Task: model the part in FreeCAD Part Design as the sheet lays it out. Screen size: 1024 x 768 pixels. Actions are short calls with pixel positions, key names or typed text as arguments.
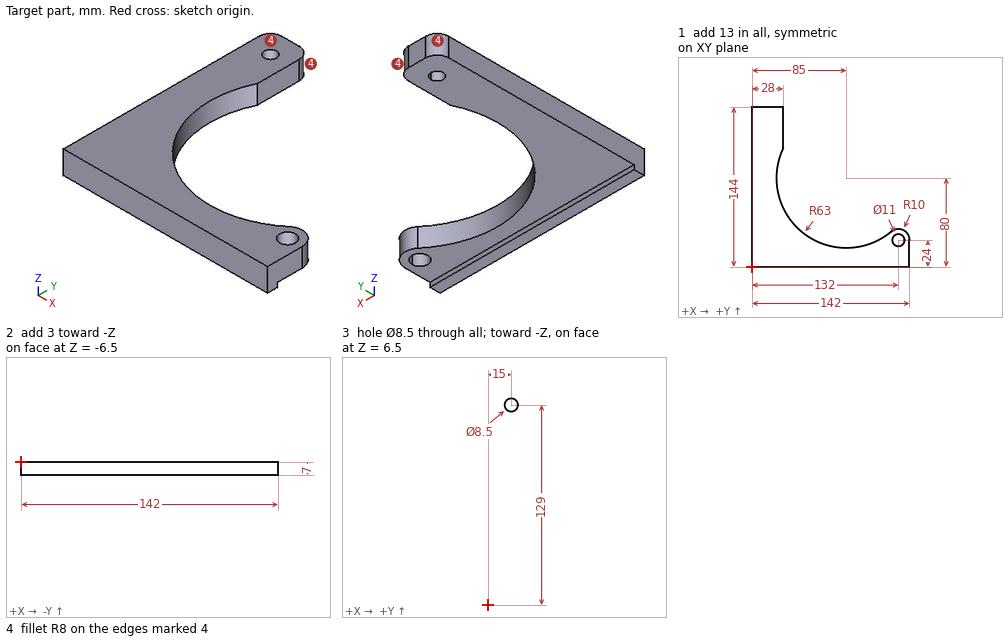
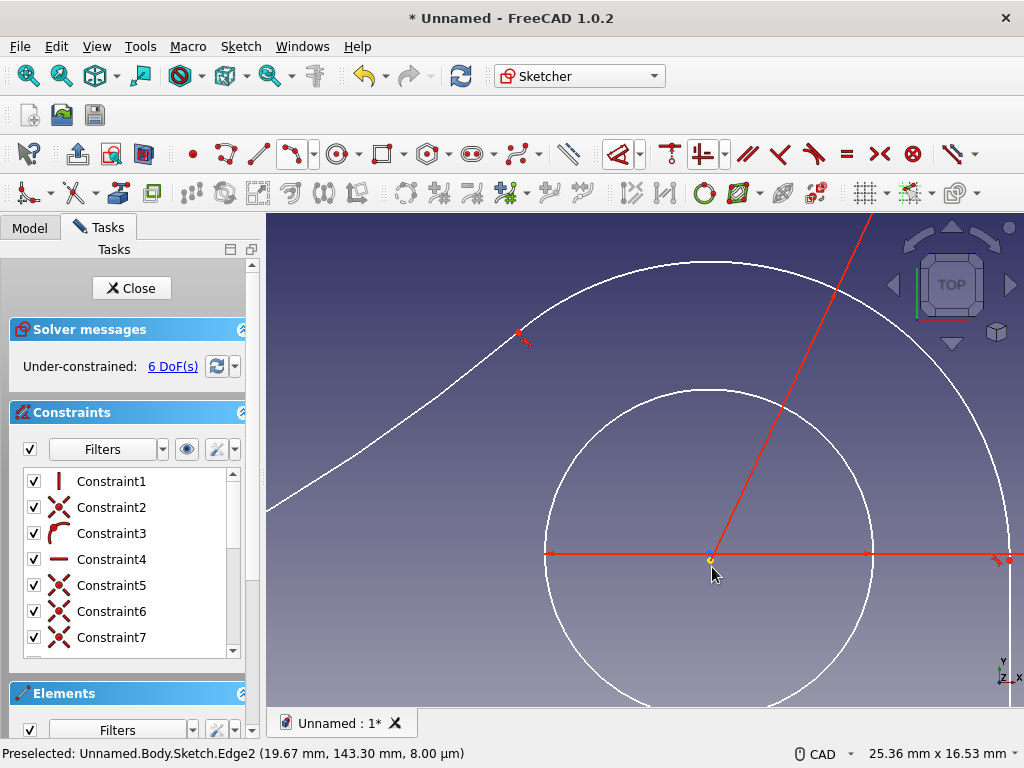
click(709, 554)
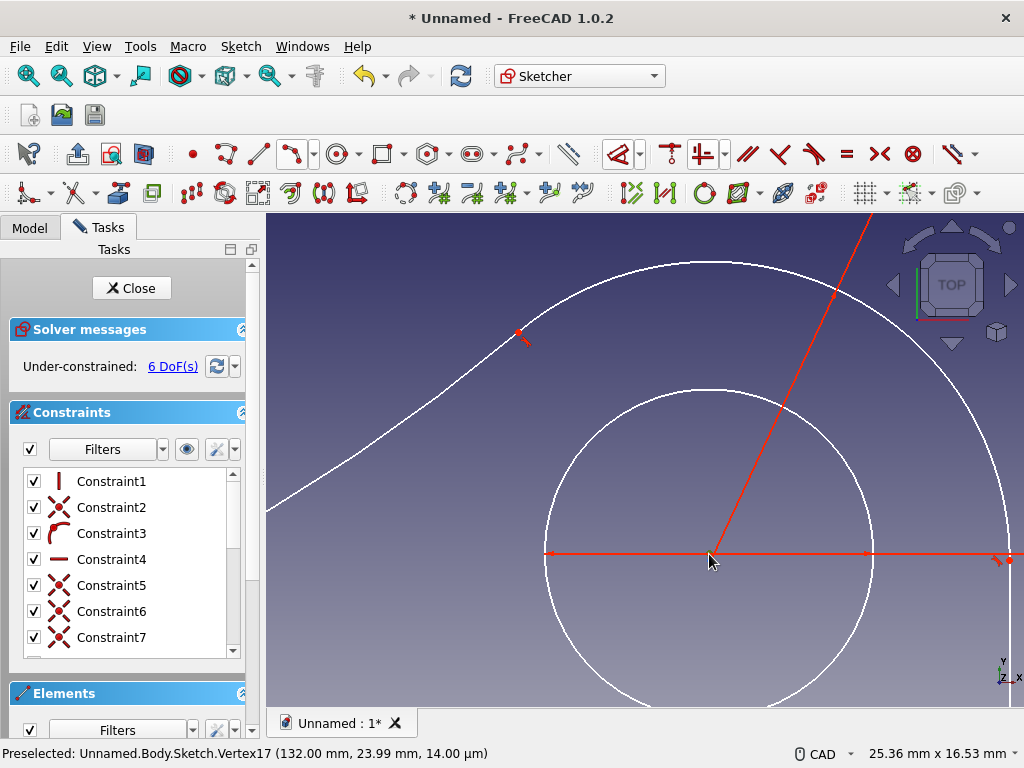
click(640, 154)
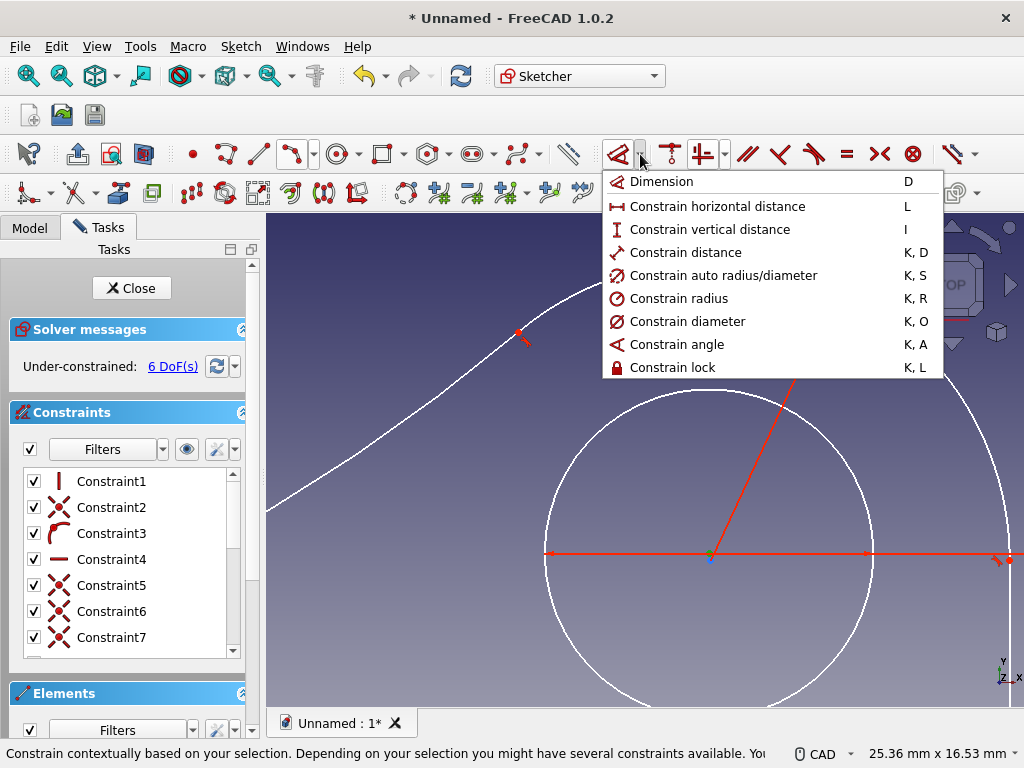
click(773, 230)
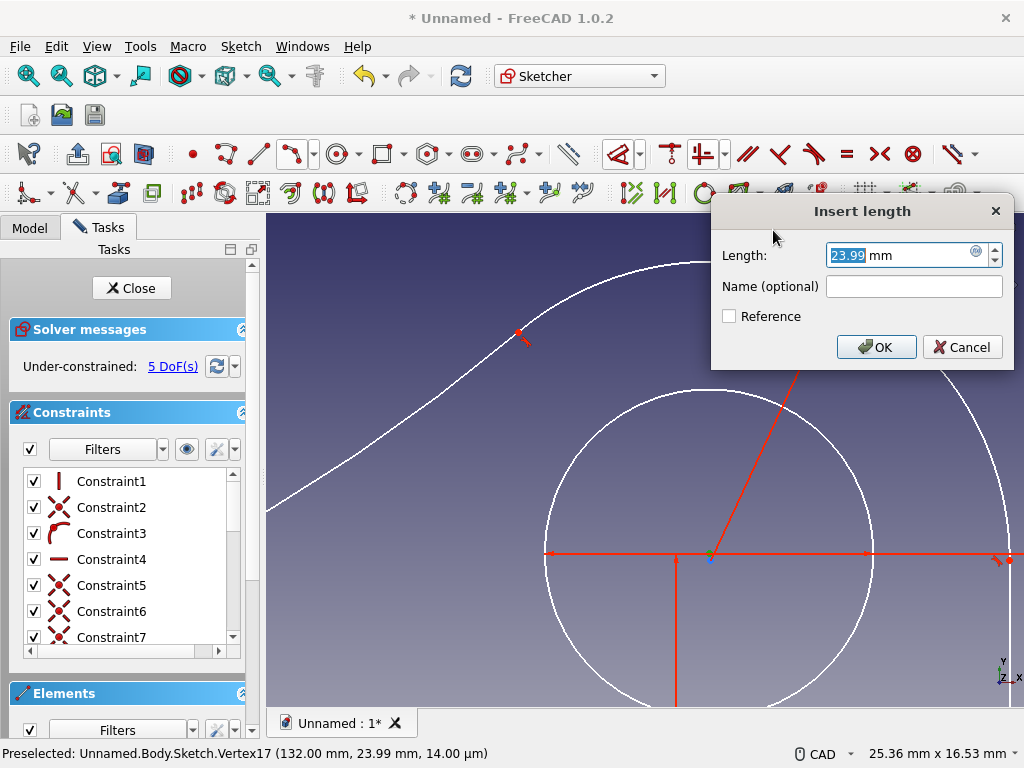
text(24)
key(Return)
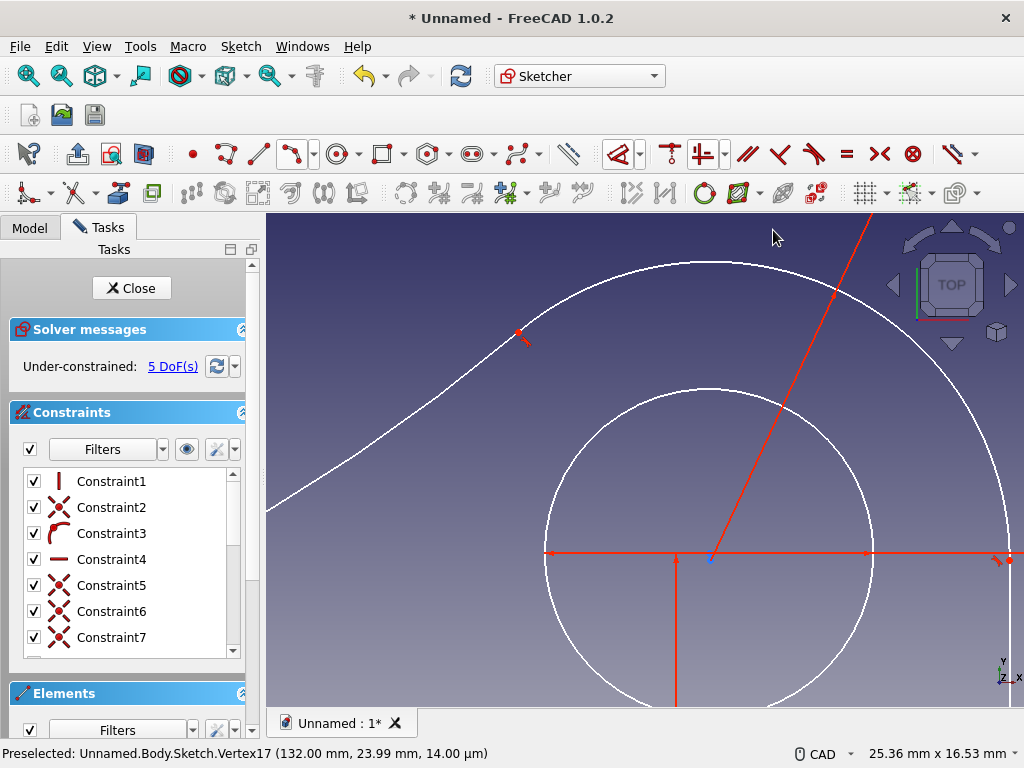
scroll(712, 568, down, 13)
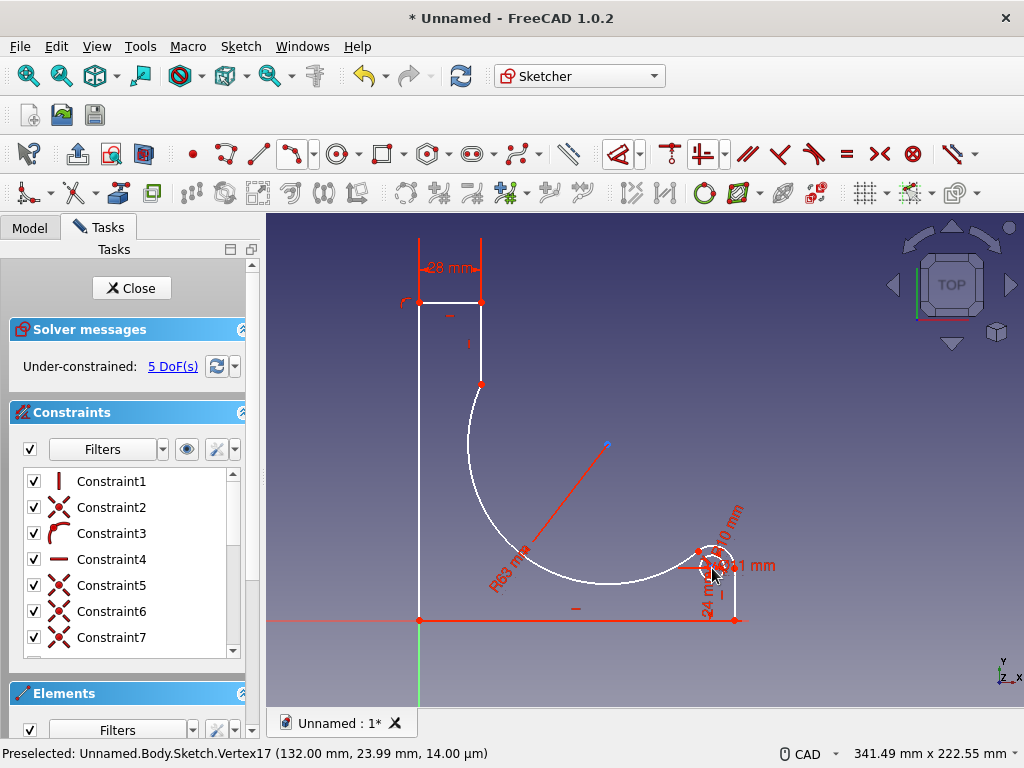
click(419, 398)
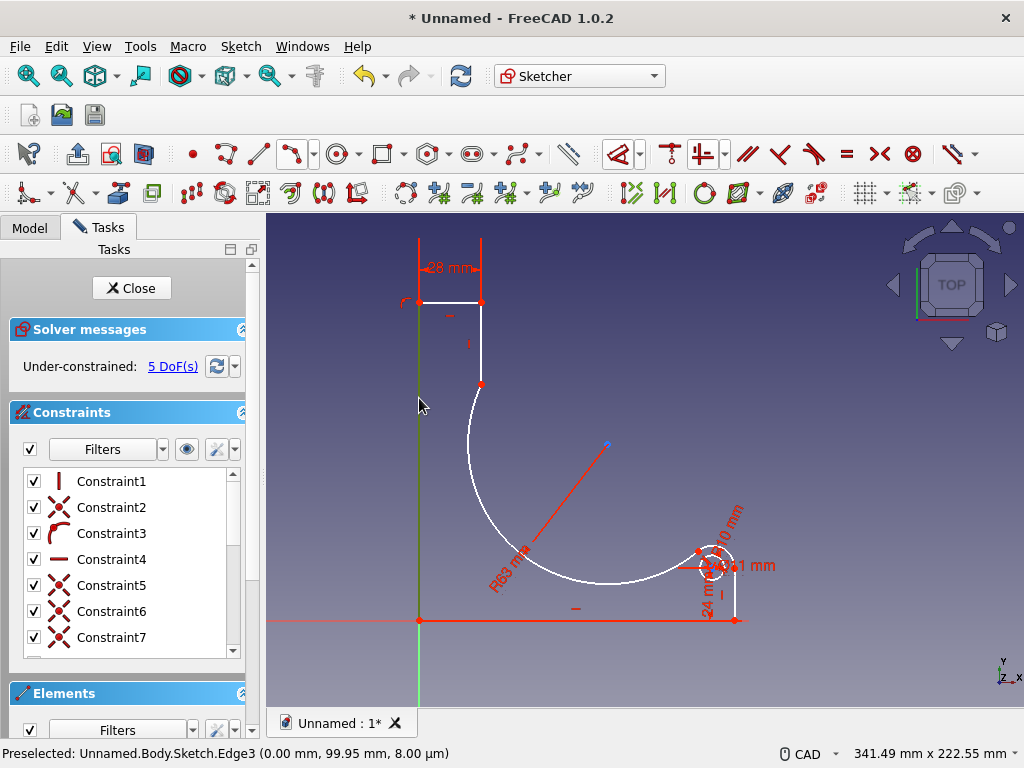
click(640, 154)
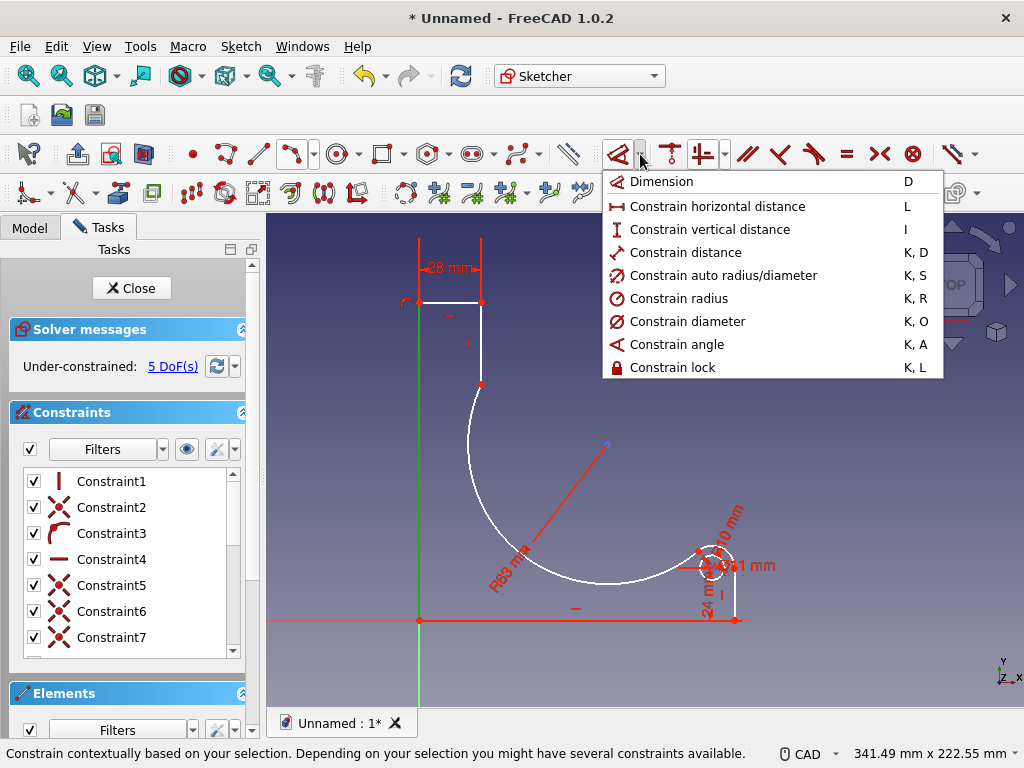
click(773, 230)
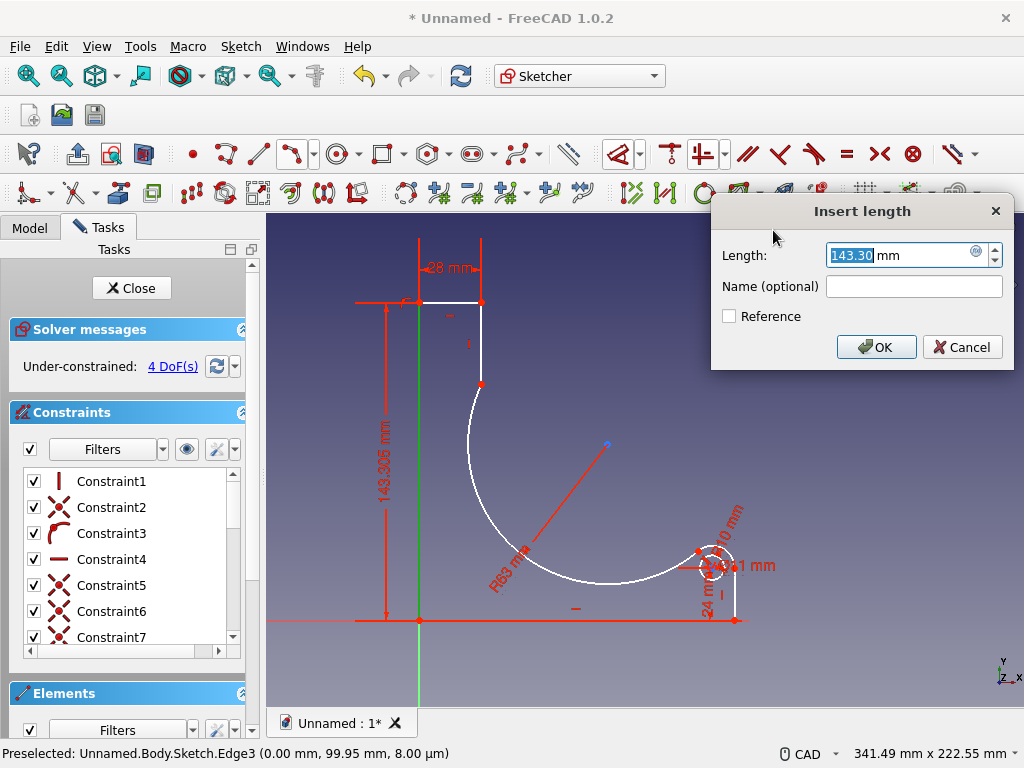
text(144)
key(Return)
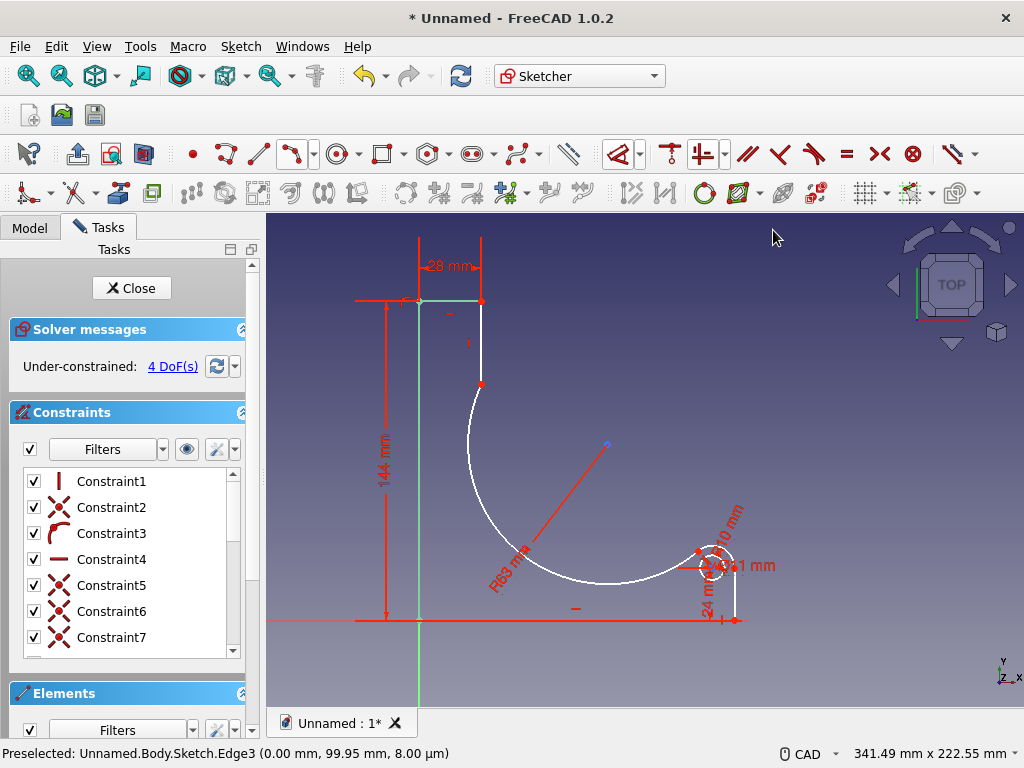
click(514, 621)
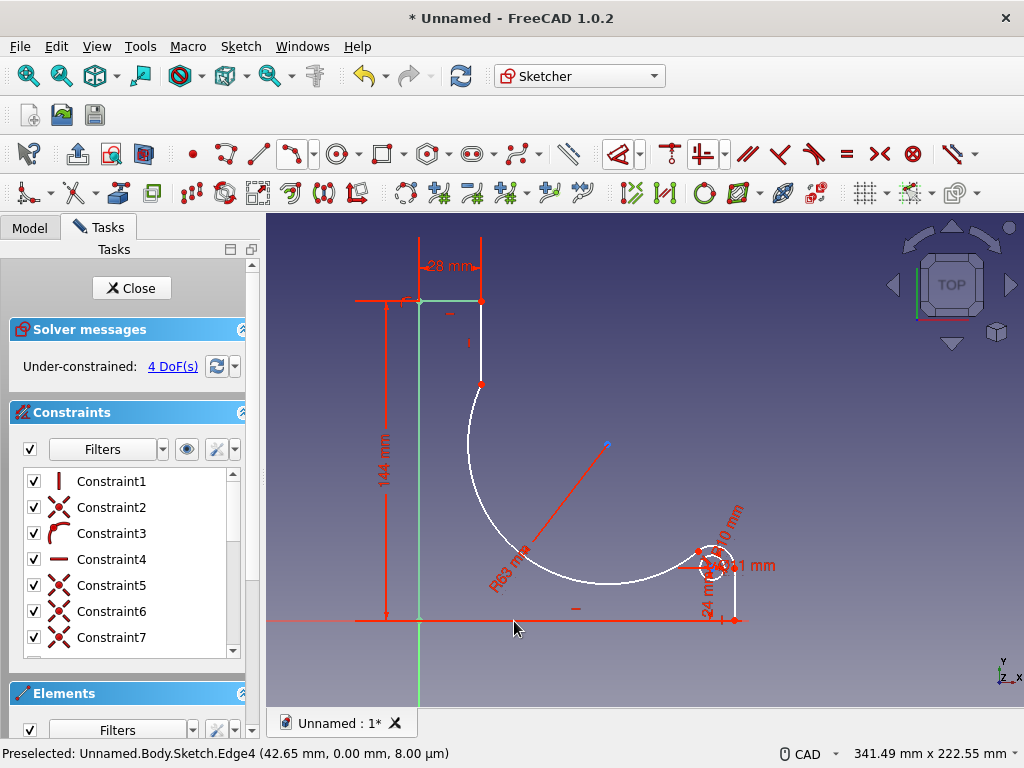
click(640, 154)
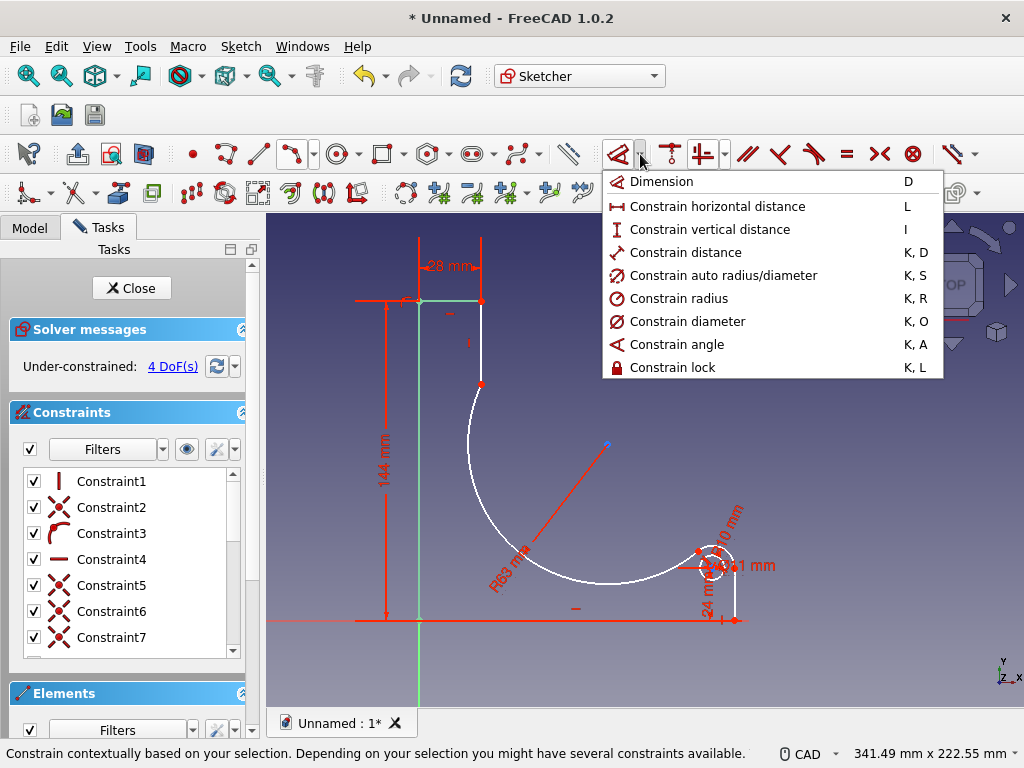
click(773, 206)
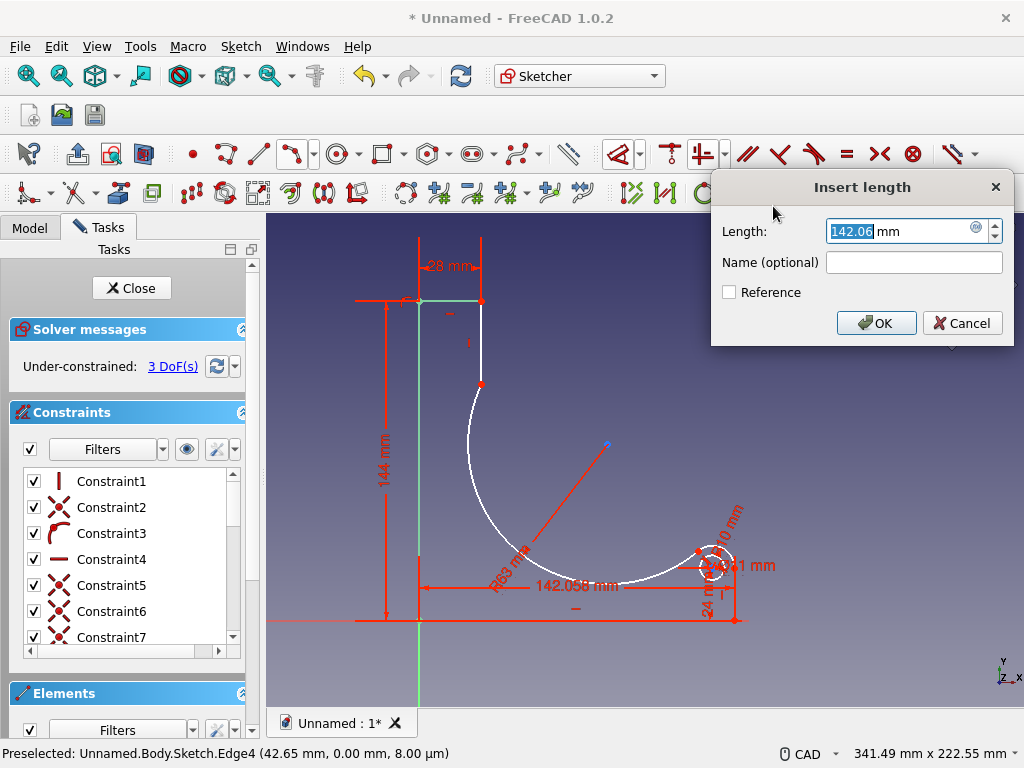
text(142)
key(Return)